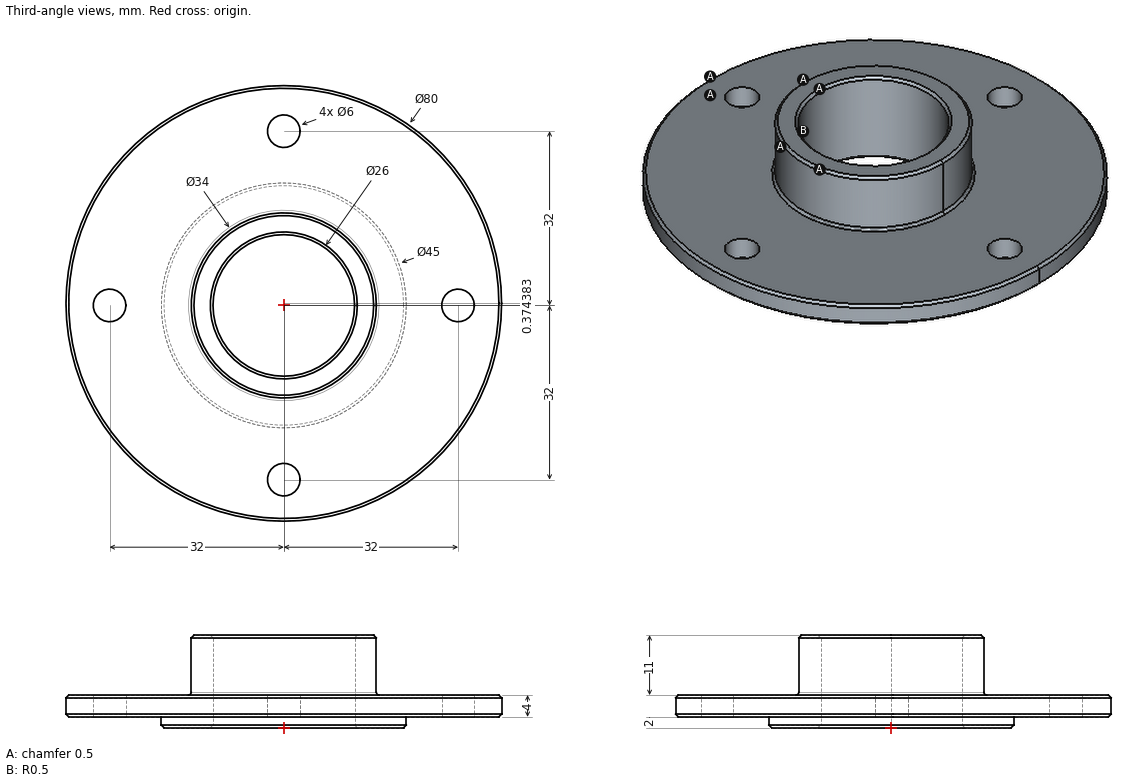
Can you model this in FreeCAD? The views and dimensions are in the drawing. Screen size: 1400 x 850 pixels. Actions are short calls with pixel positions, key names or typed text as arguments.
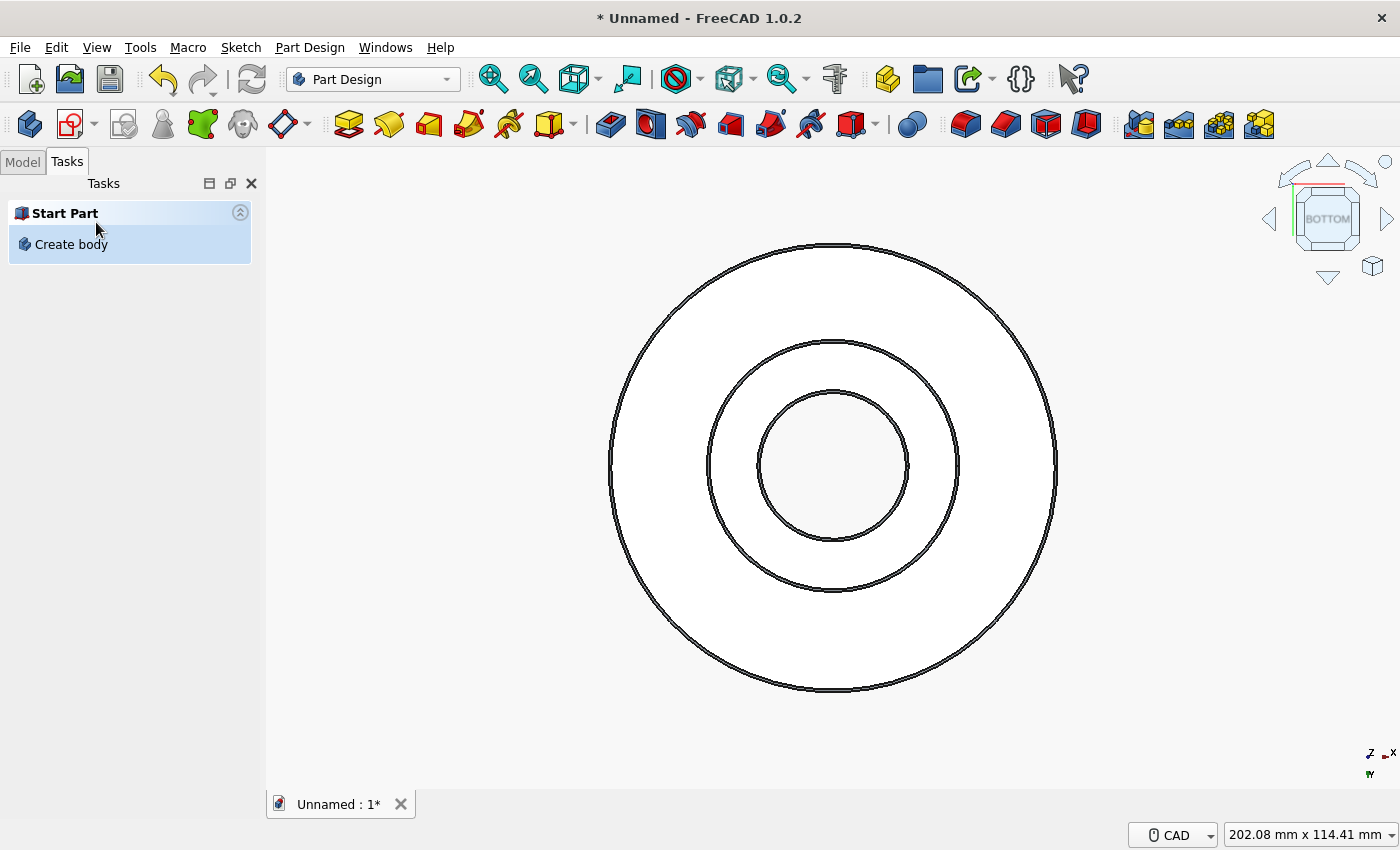
key(0)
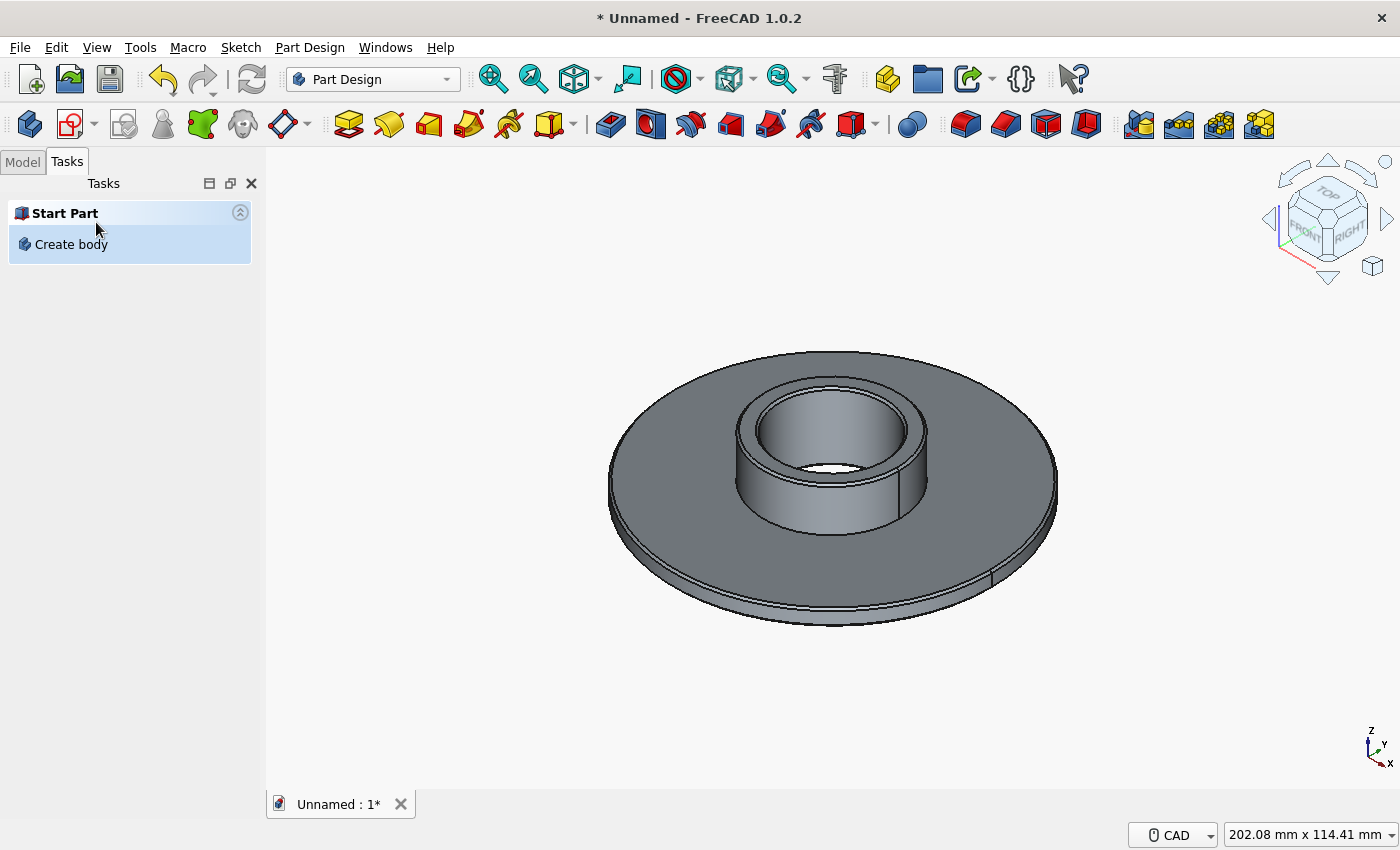
key(2)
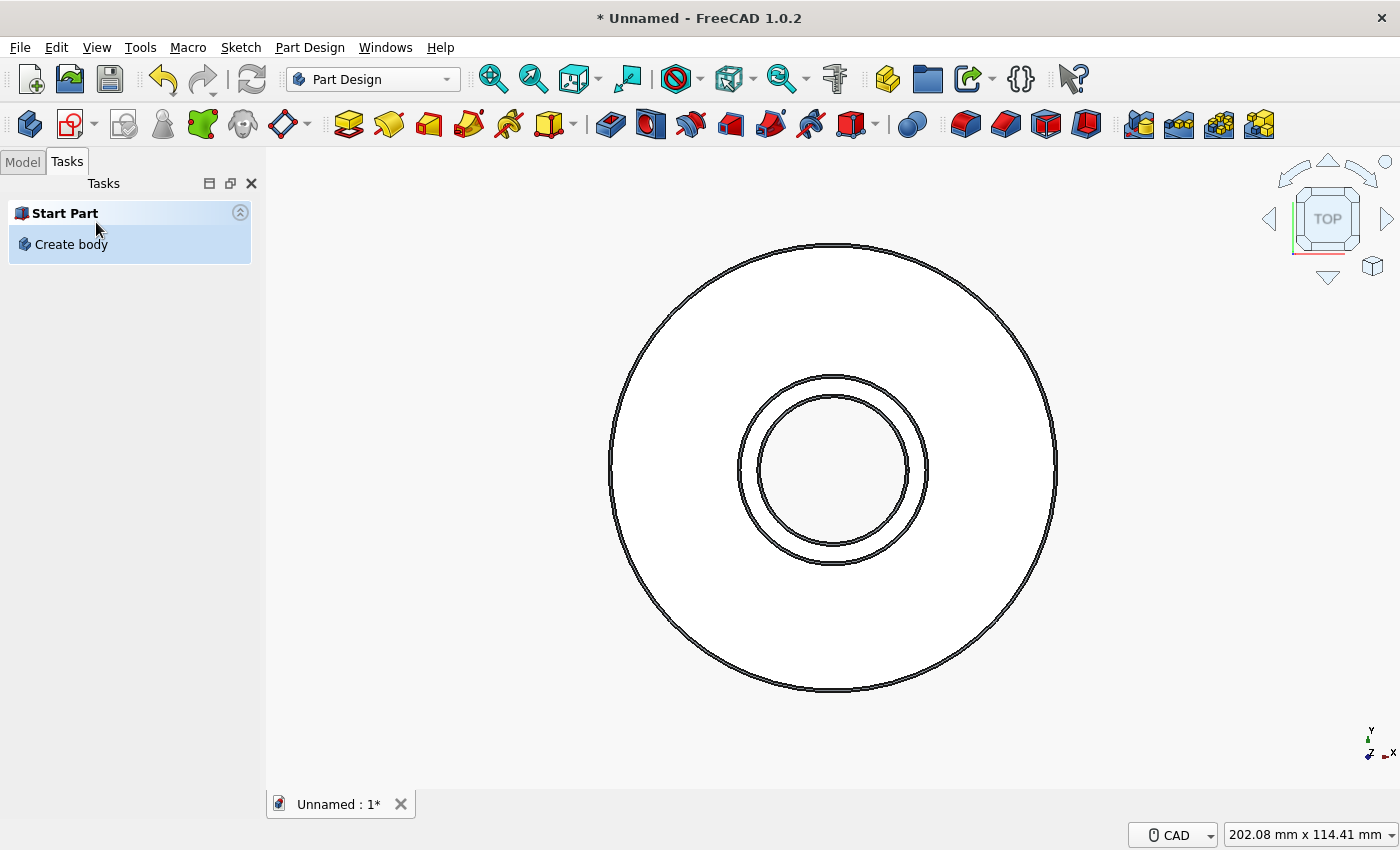
key(1)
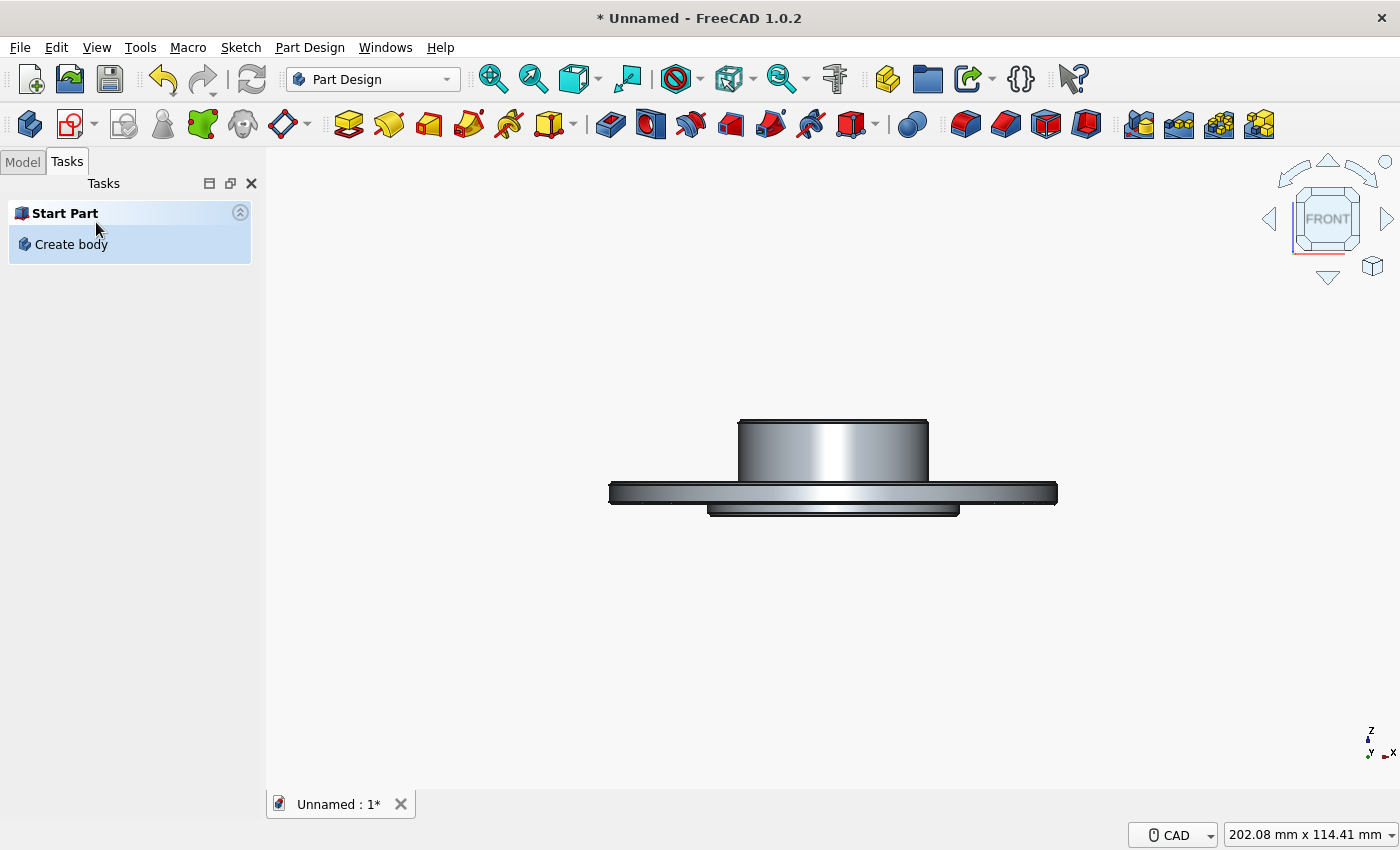
click(494, 80)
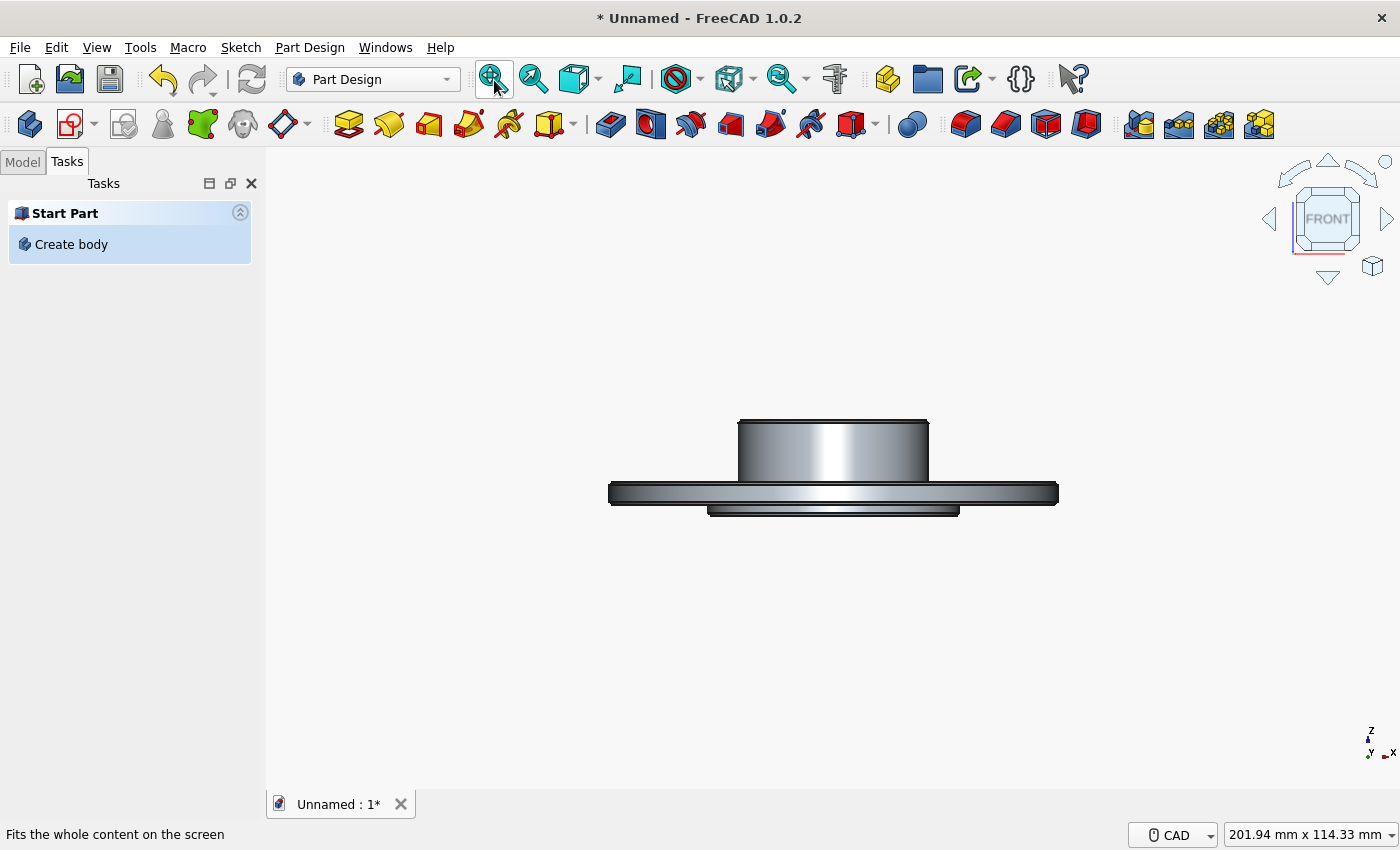
key(3)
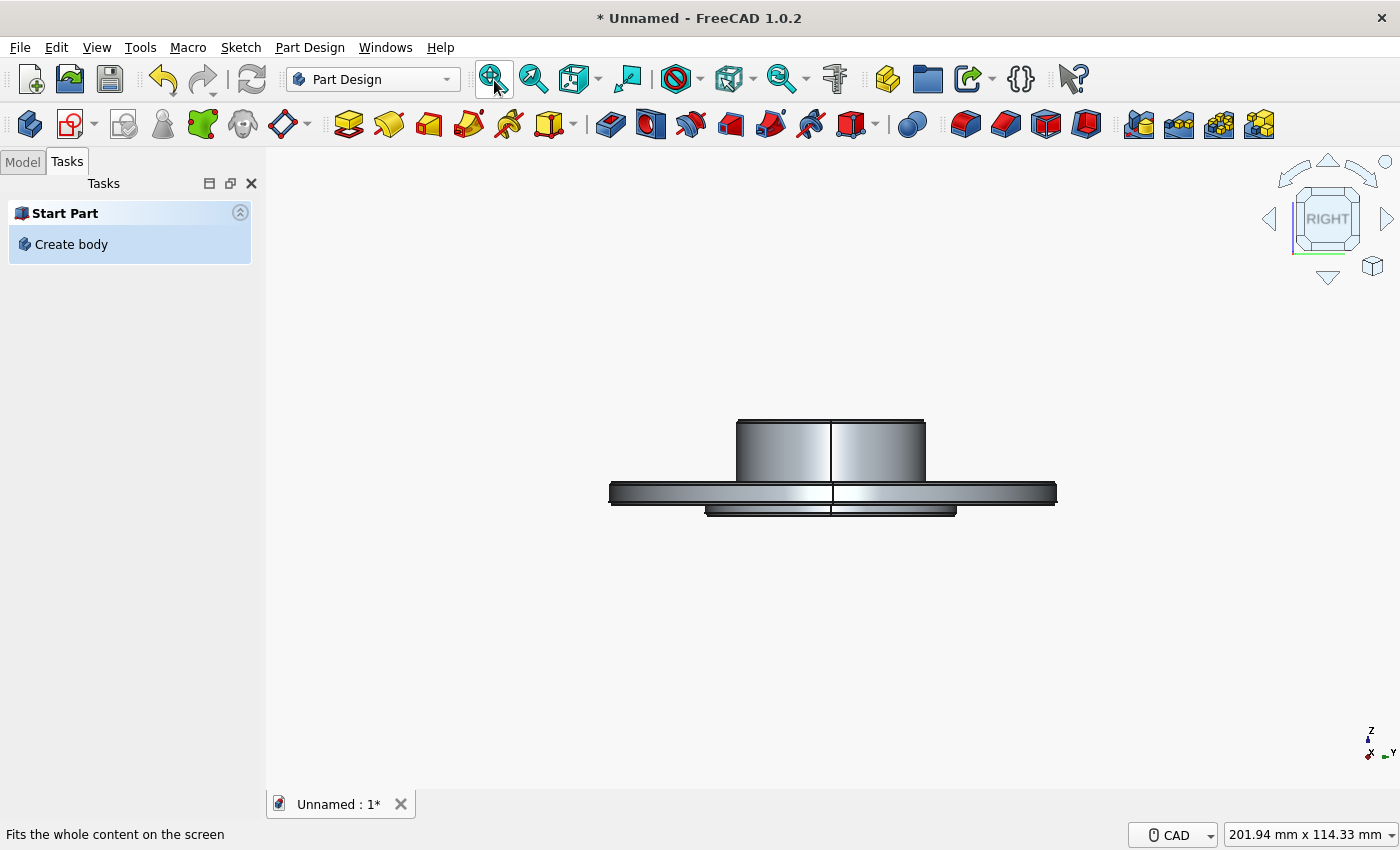
click(494, 80)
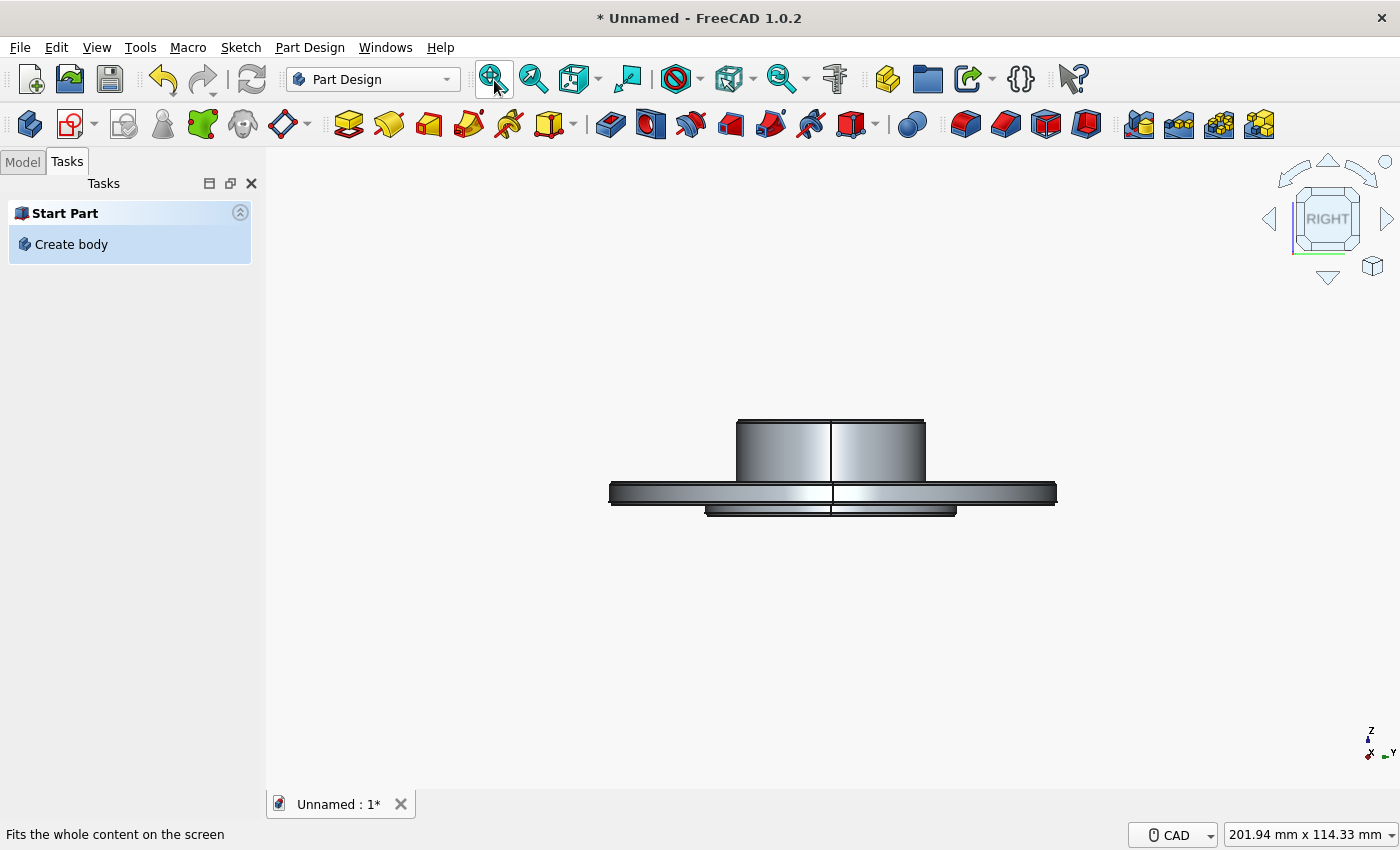
key(5)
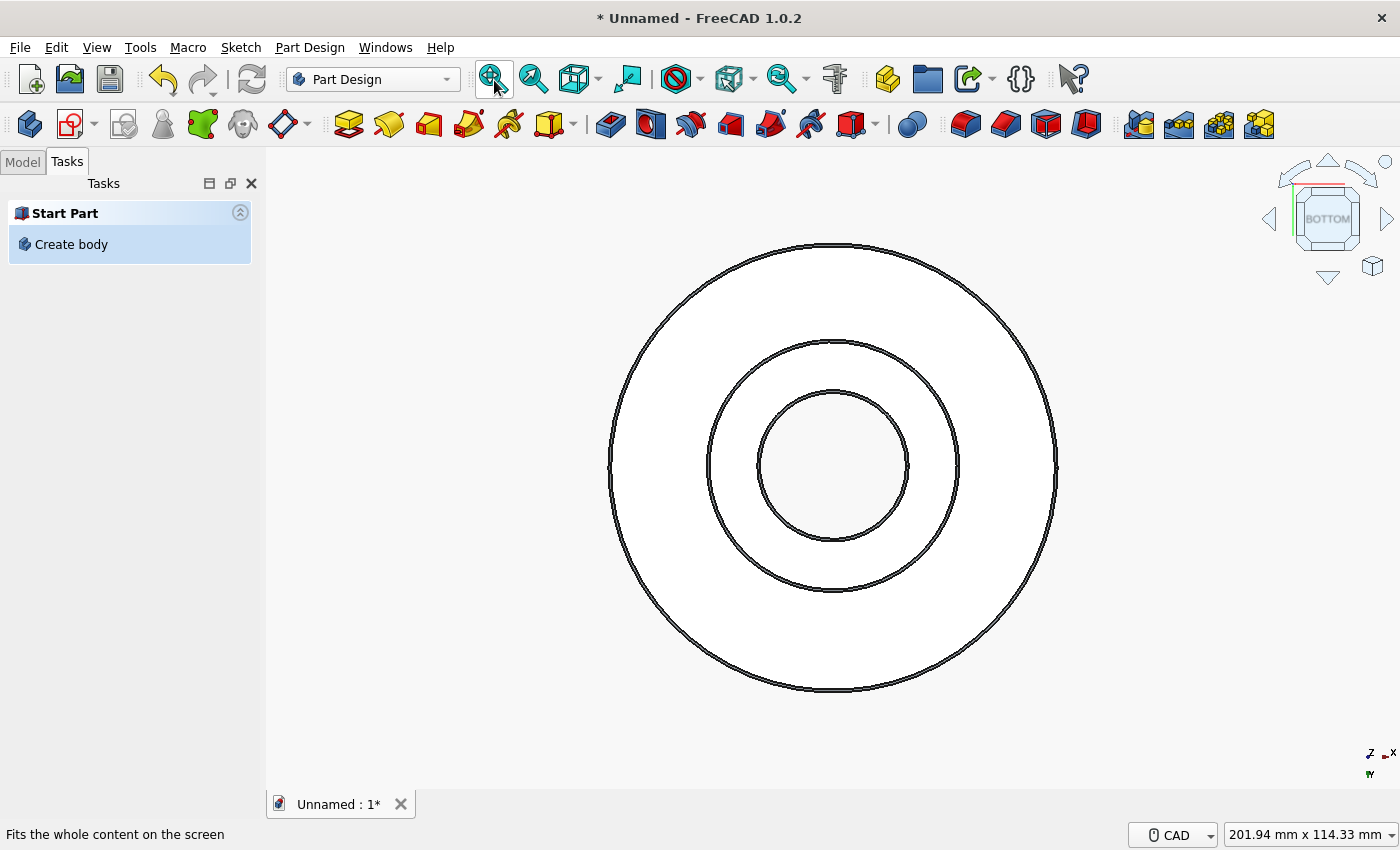
key(4)